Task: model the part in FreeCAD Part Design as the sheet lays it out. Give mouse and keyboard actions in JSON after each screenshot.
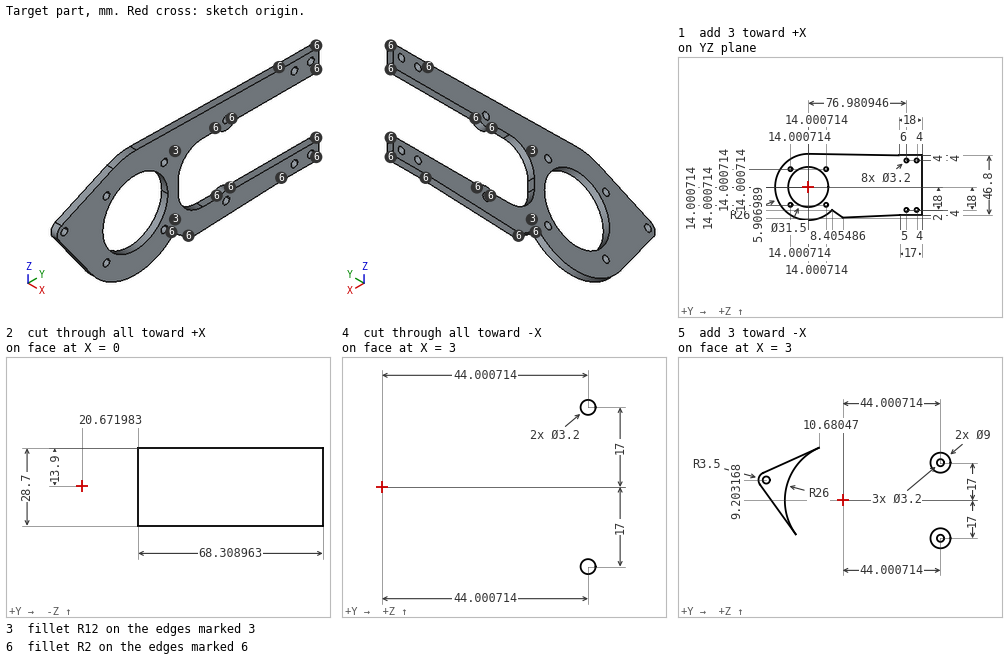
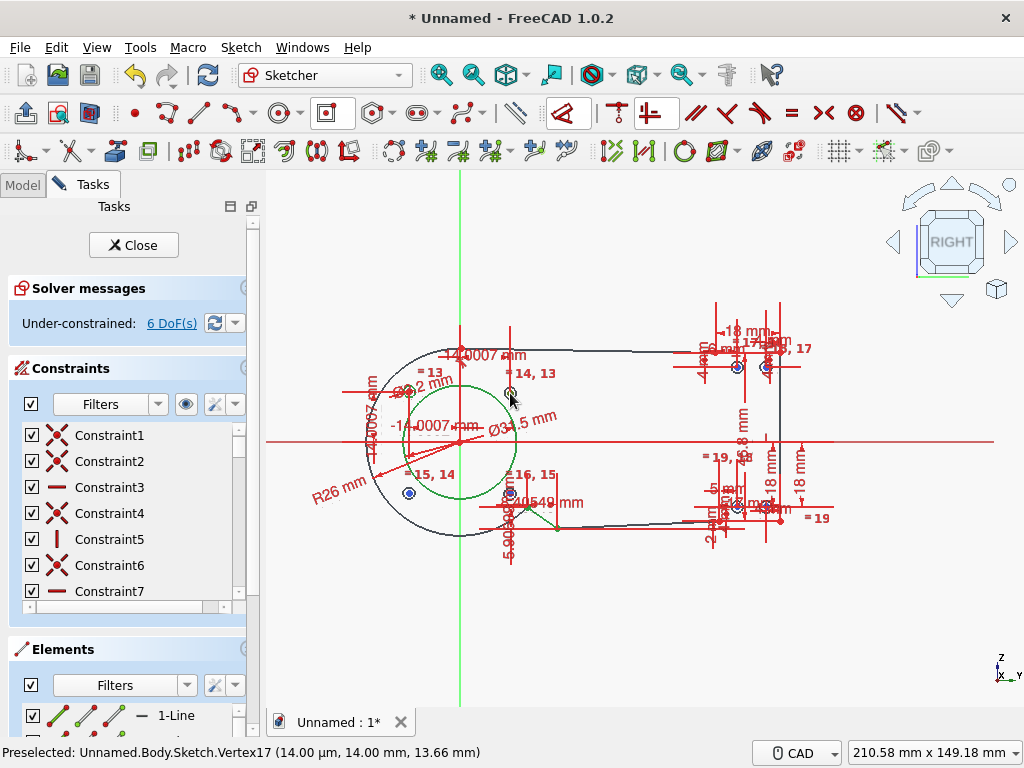
{"action": "key", "text": "i"}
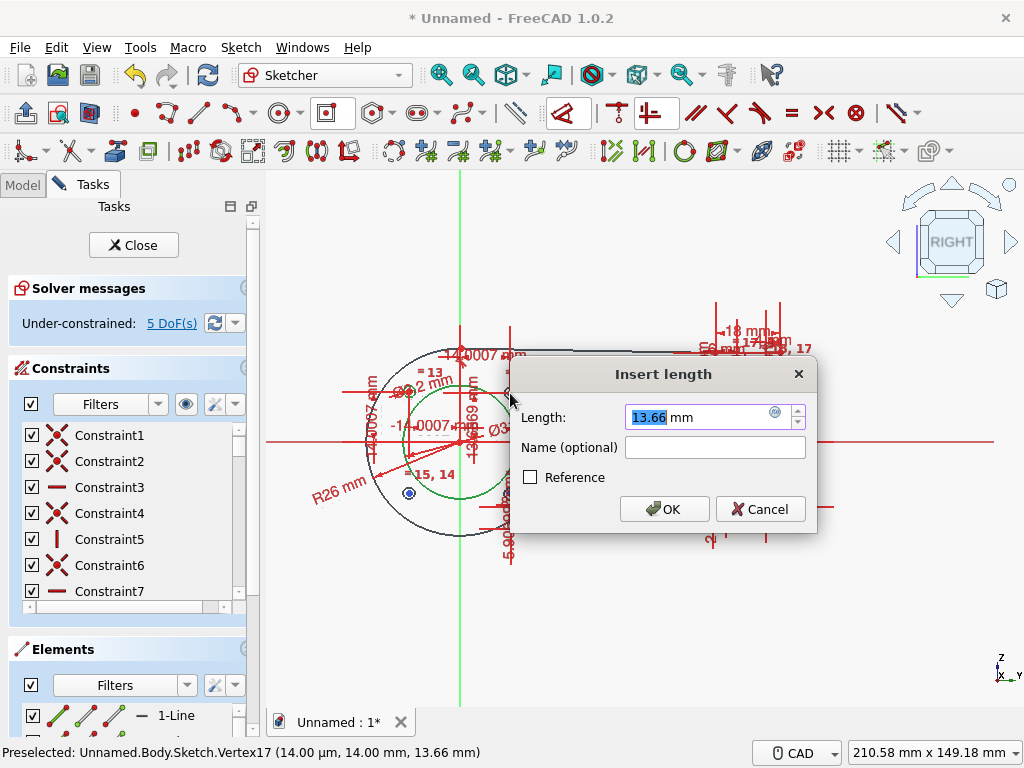
{"action": "type", "text": "14.000714"}
{"action": "key", "text": "Return"}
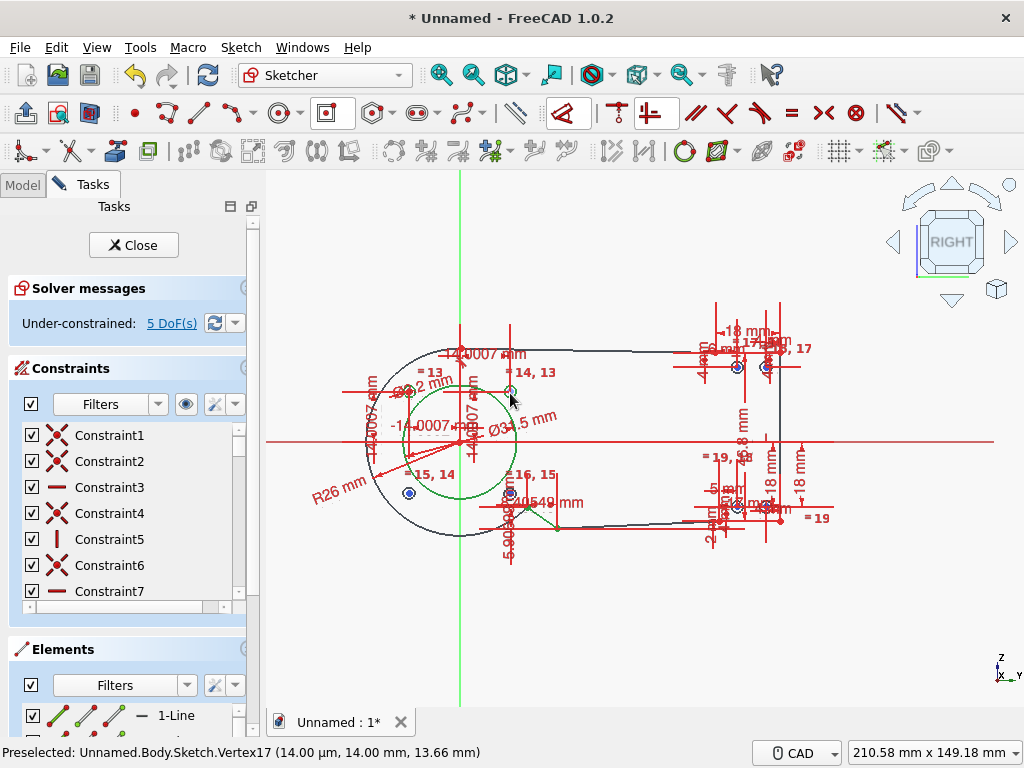
{"action": "left_click", "coordinate": [409, 493]}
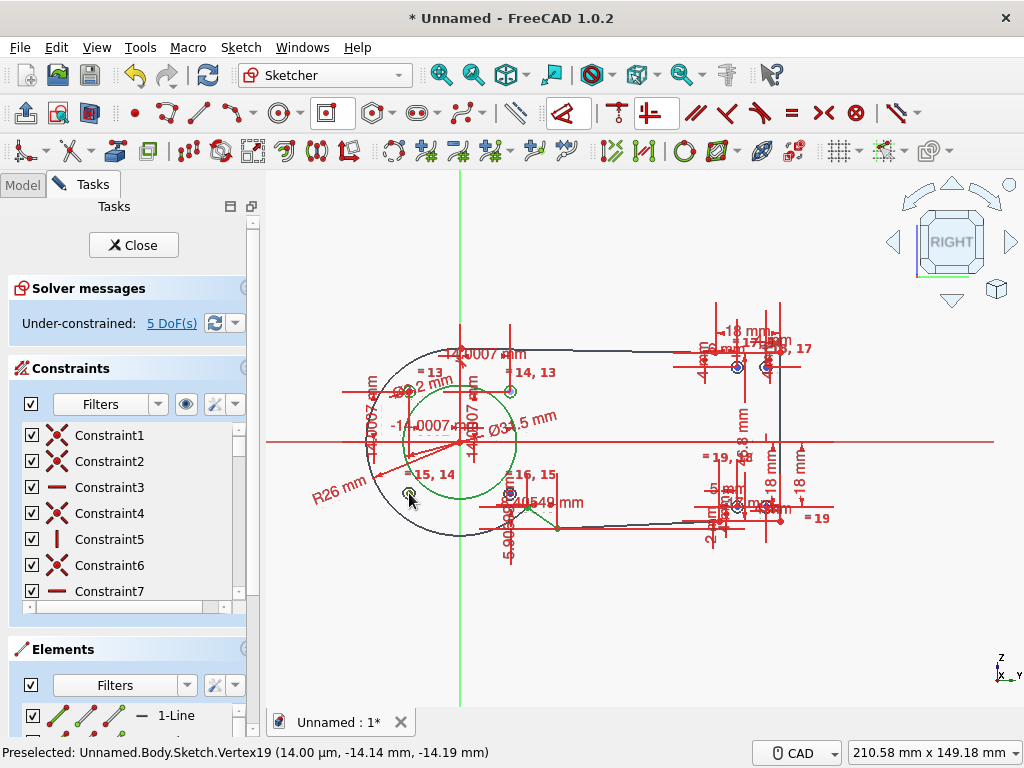
{"action": "left_click", "coordinate": [586, 114]}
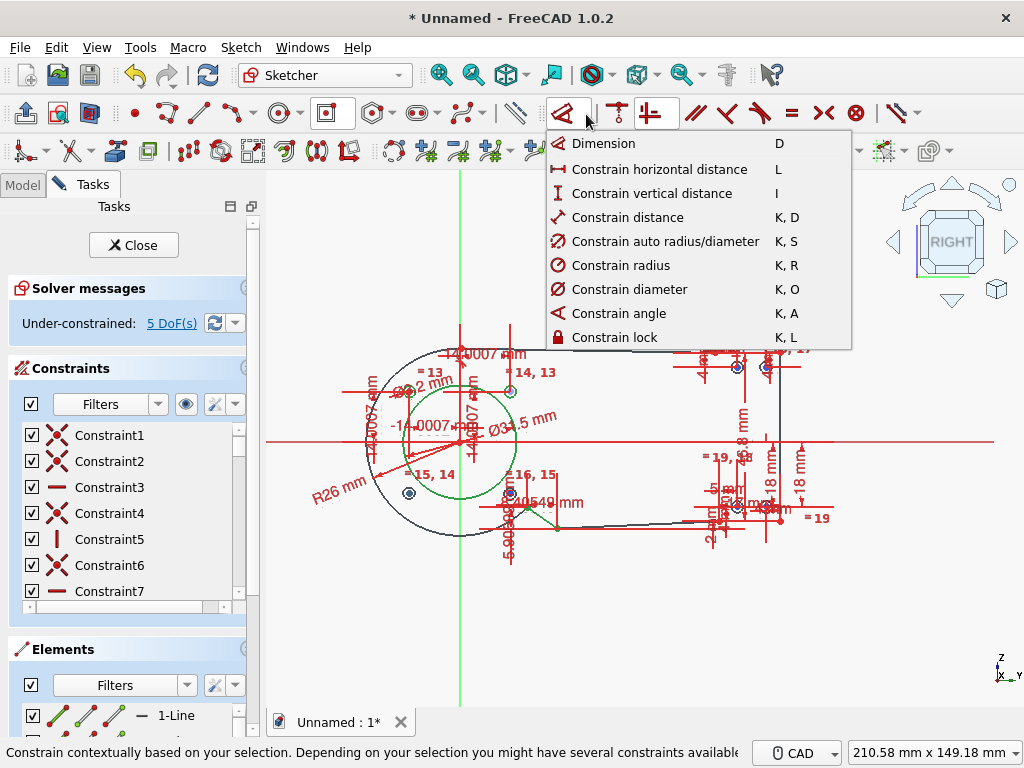
{"action": "left_click", "coordinate": [699, 169]}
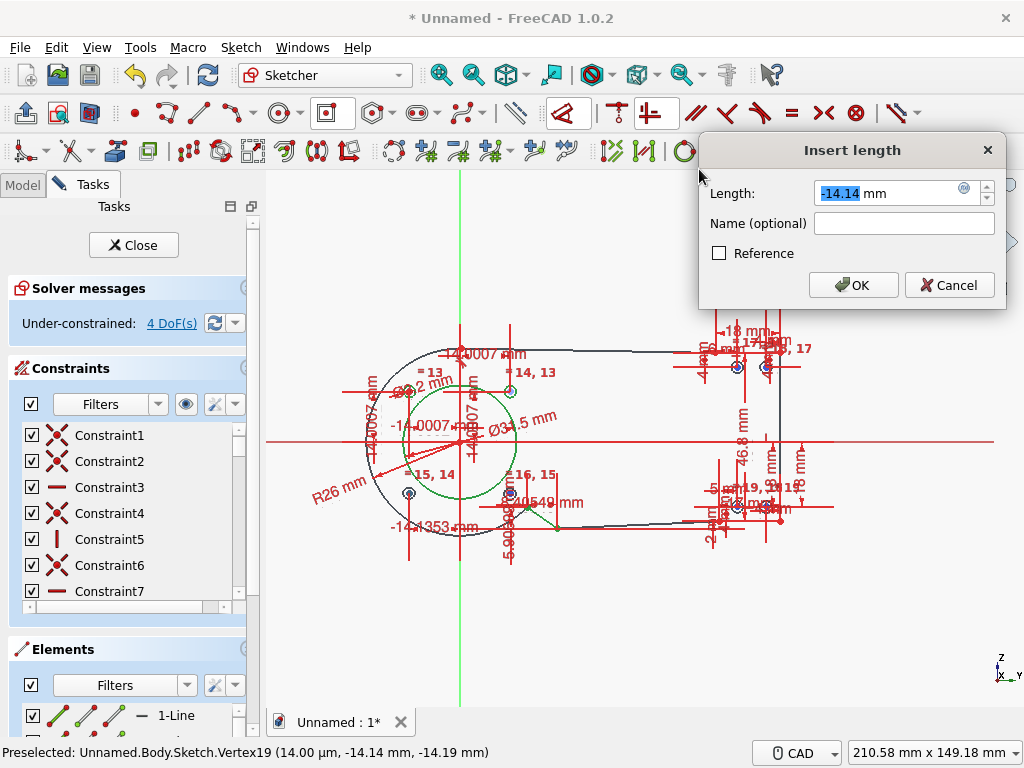
{"action": "type", "text": "-14.000714"}
{"action": "key", "text": "Return"}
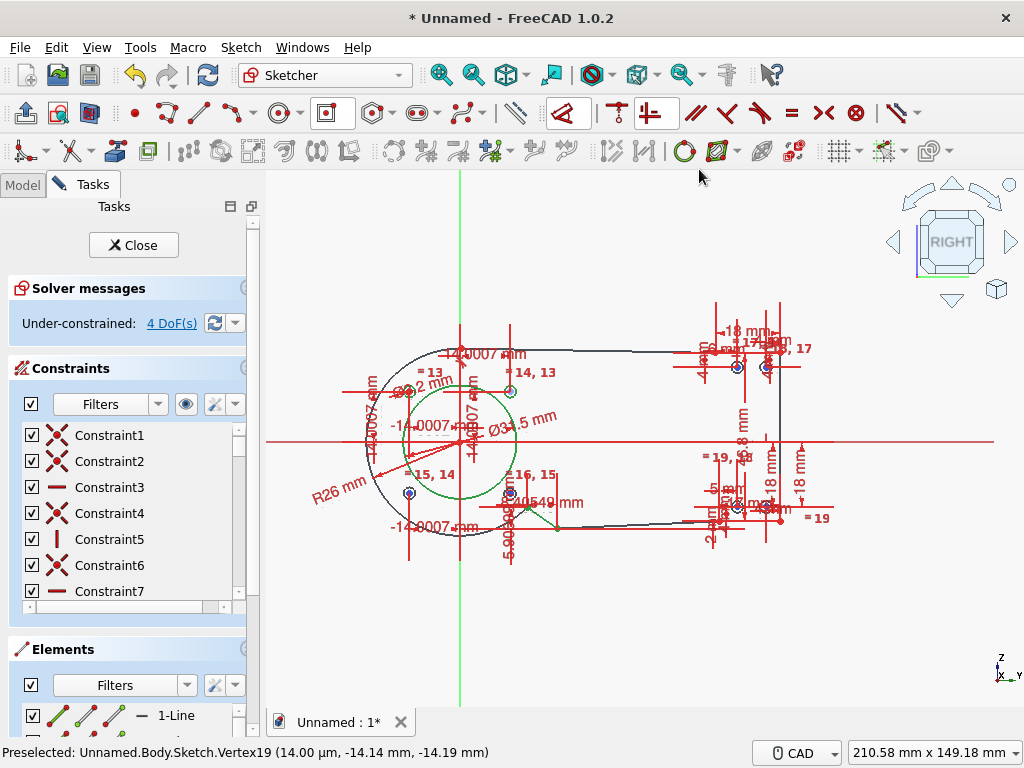
{"action": "left_click", "coordinate": [409, 493]}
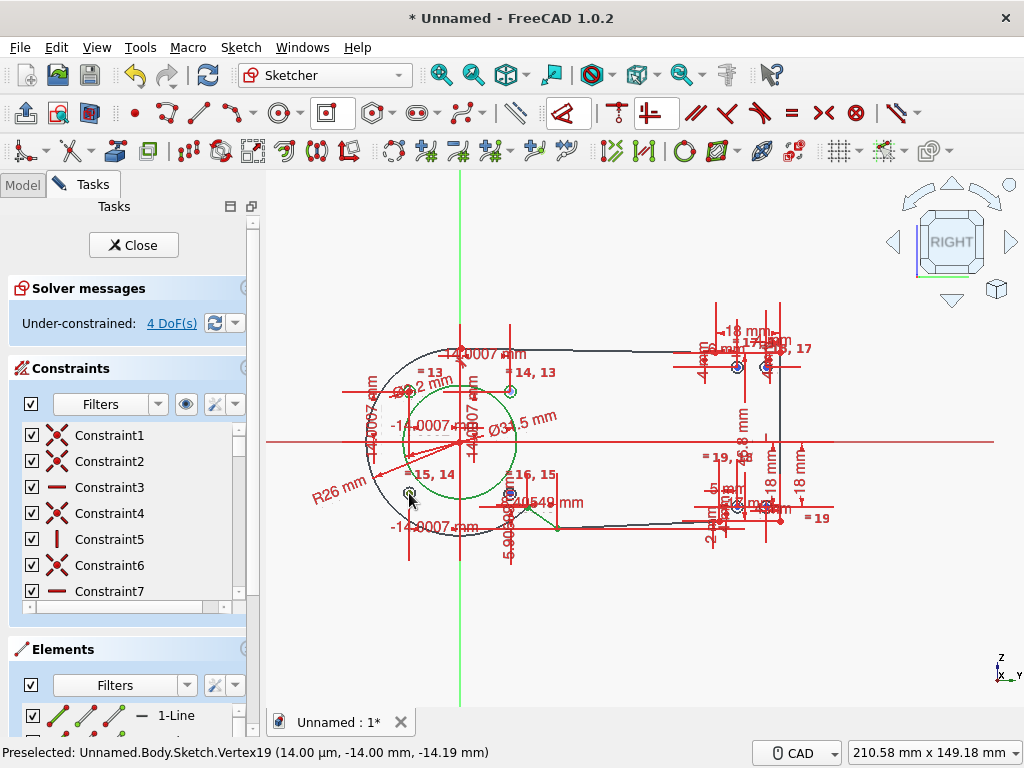
{"action": "left_click", "coordinate": [586, 114]}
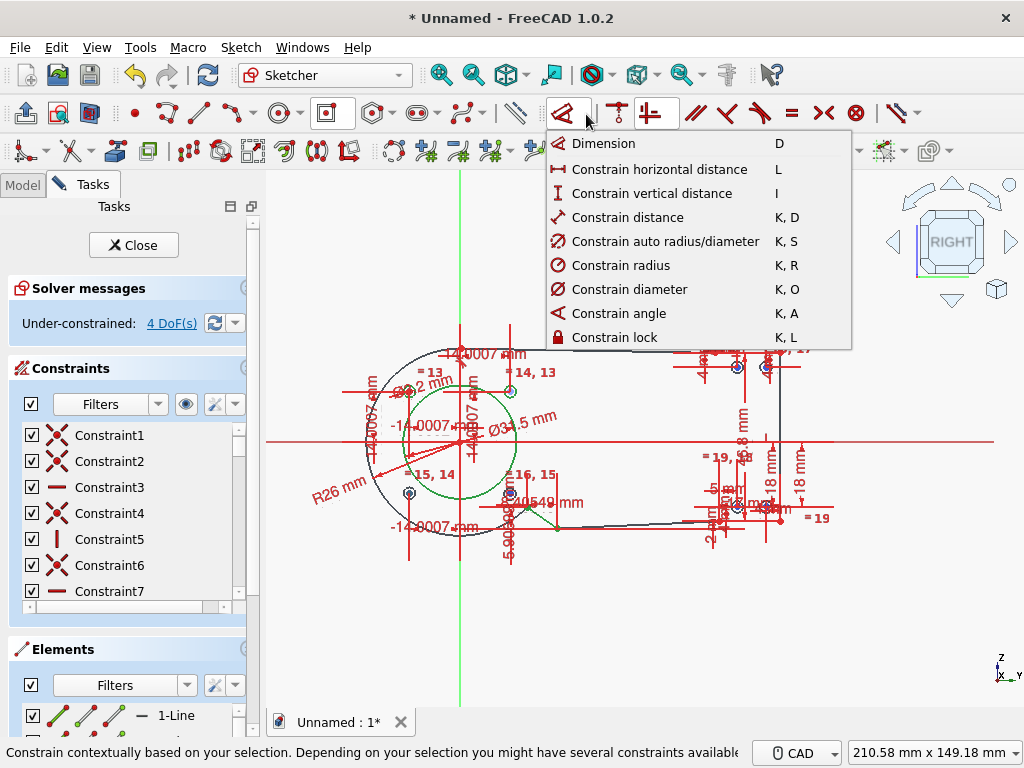
{"action": "left_click", "coordinate": [699, 193]}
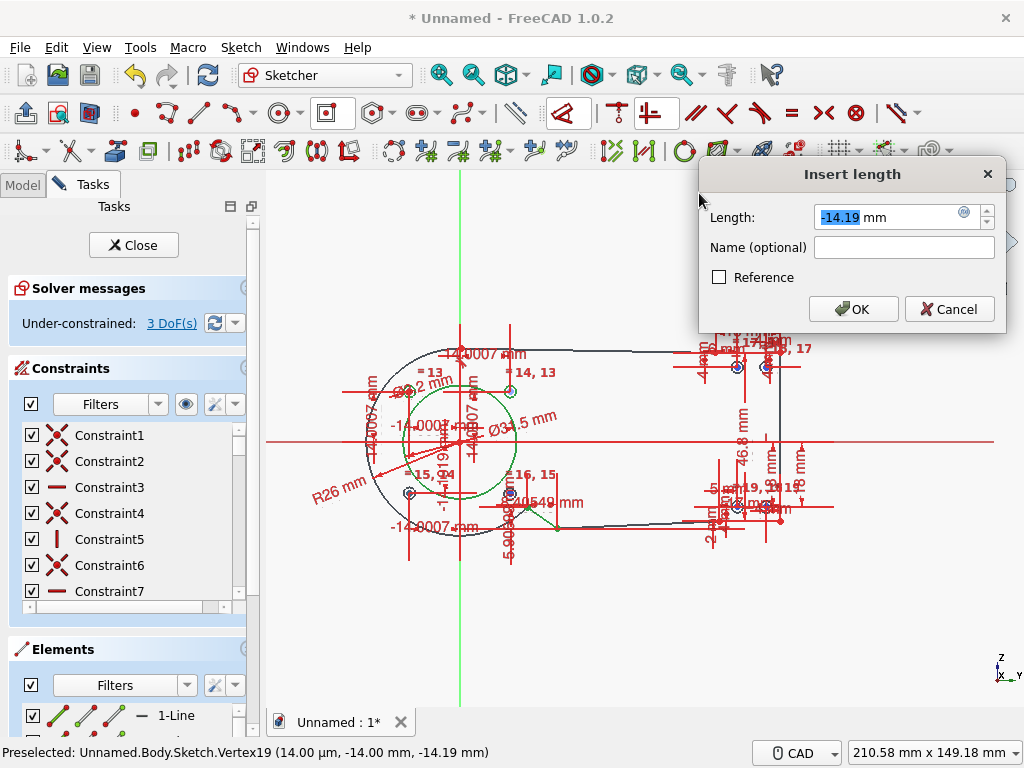
{"action": "type", "text": "-14.000714"}
{"action": "key", "text": "Return"}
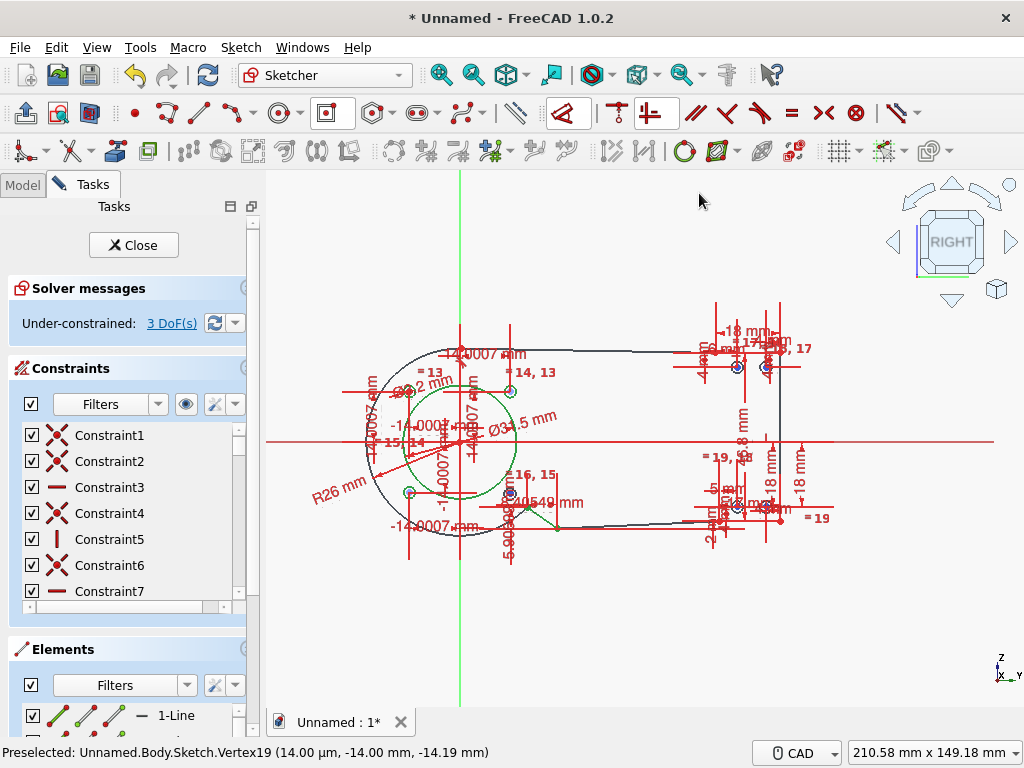
{"action": "left_click", "coordinate": [510, 494]}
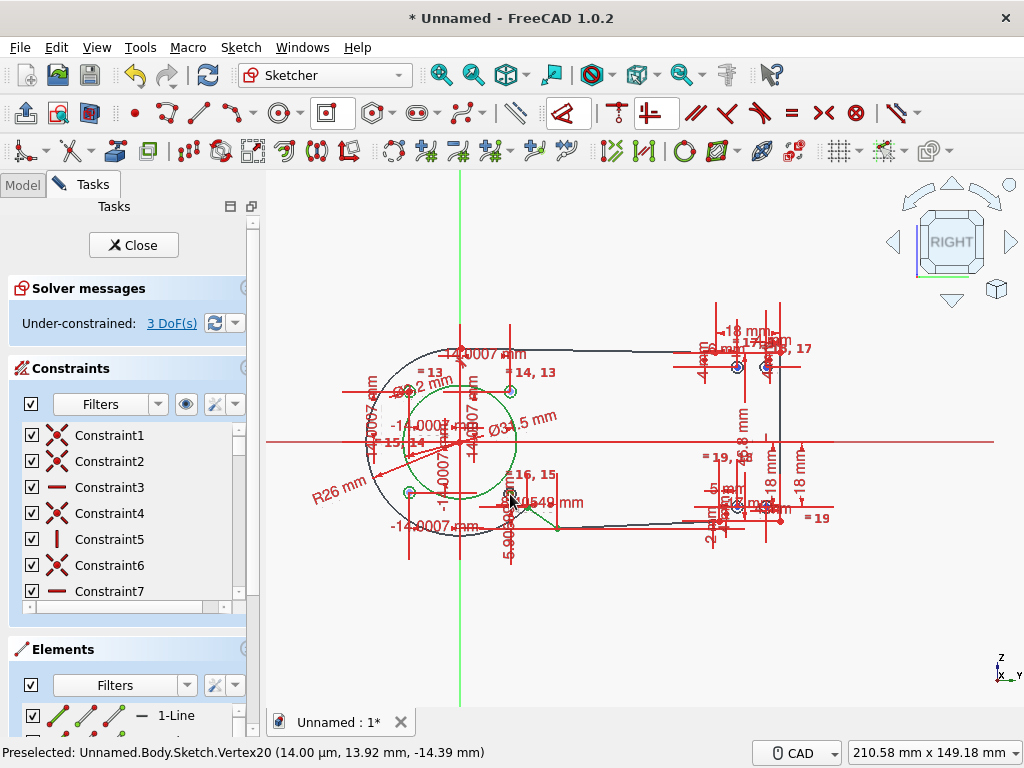
{"action": "key", "text": "l"}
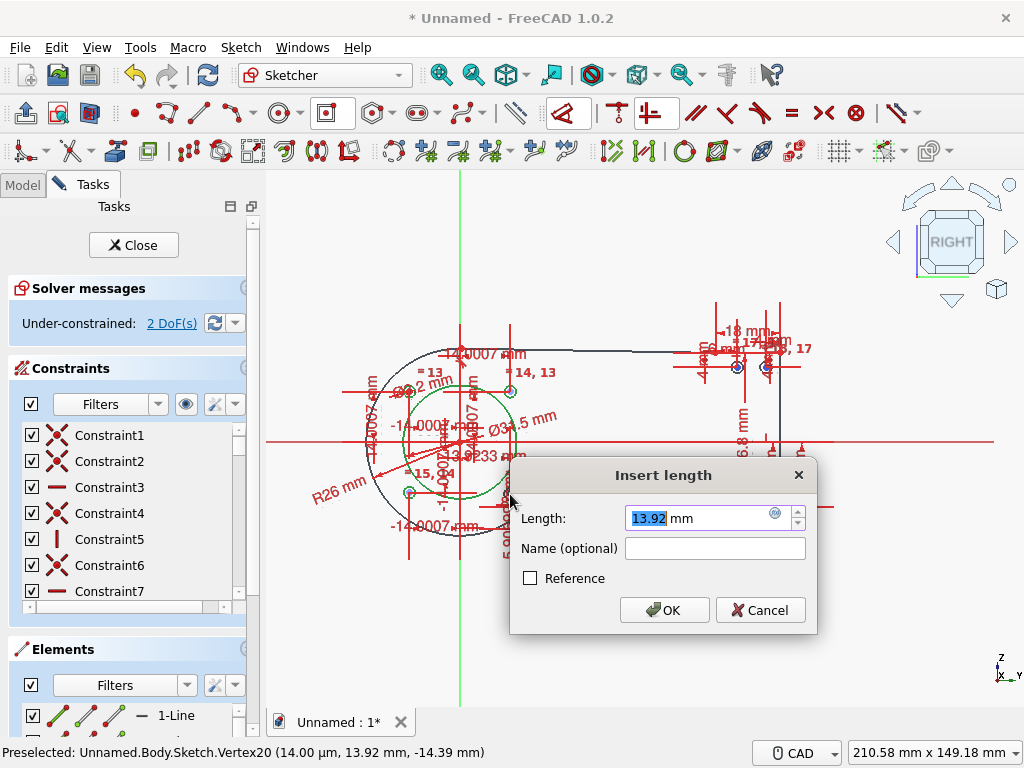
{"action": "type", "text": "14.000714"}
{"action": "key", "text": "Return"}